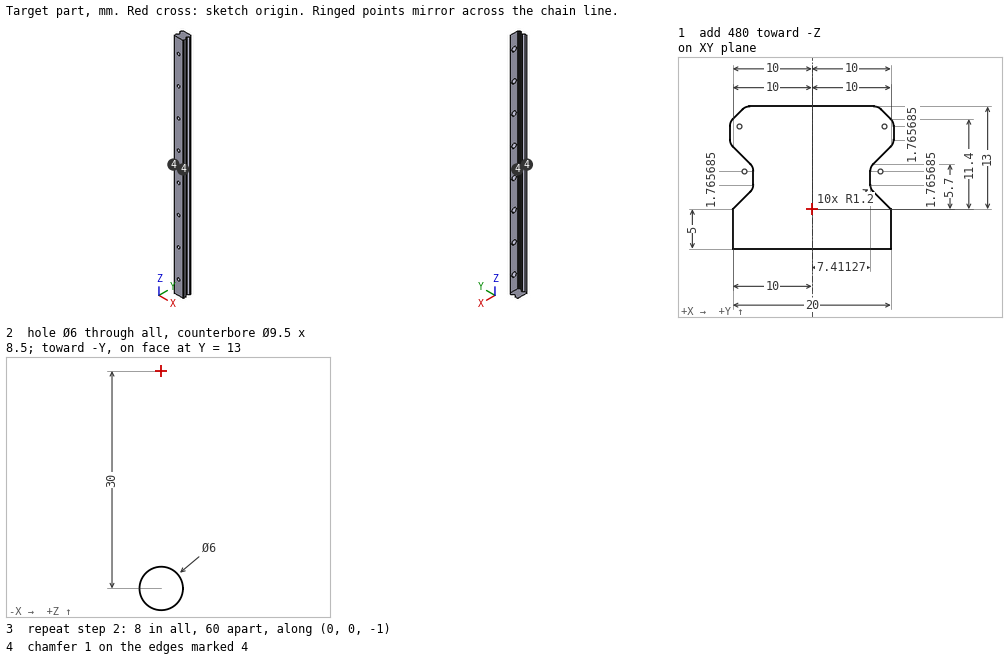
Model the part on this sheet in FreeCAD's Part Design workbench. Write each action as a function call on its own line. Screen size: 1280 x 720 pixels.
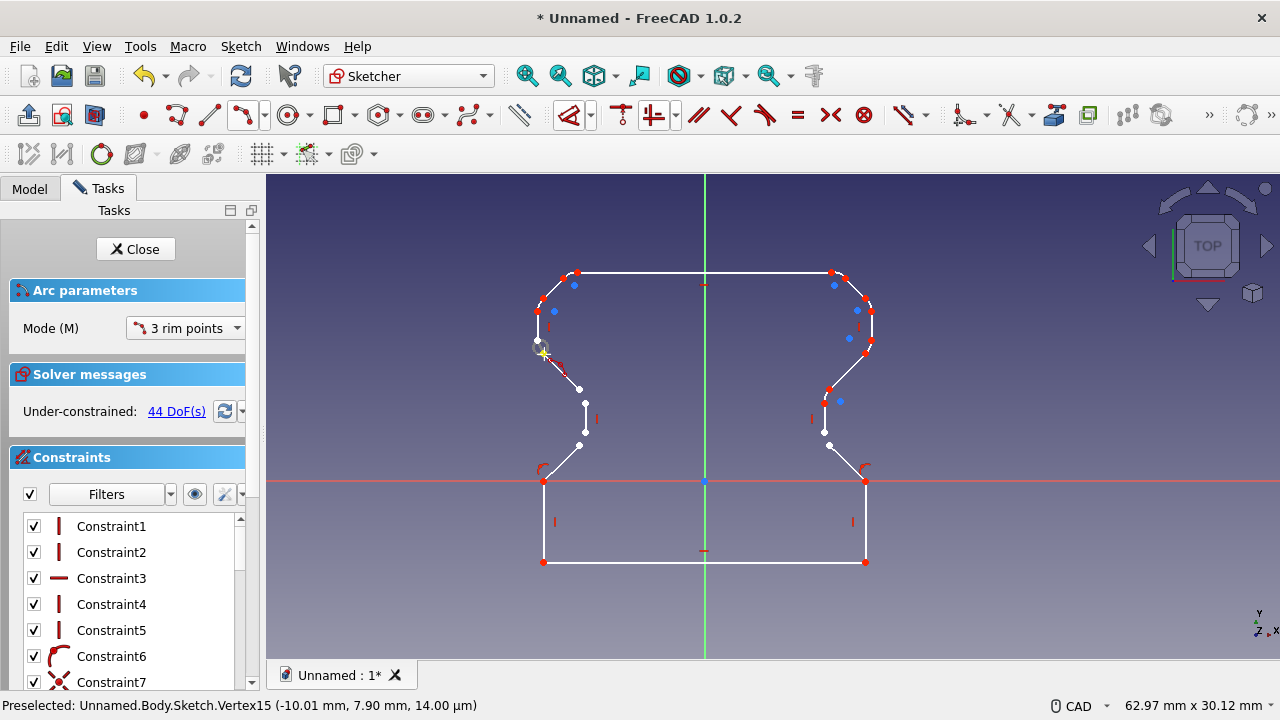
scroll(540, 347, up, 12)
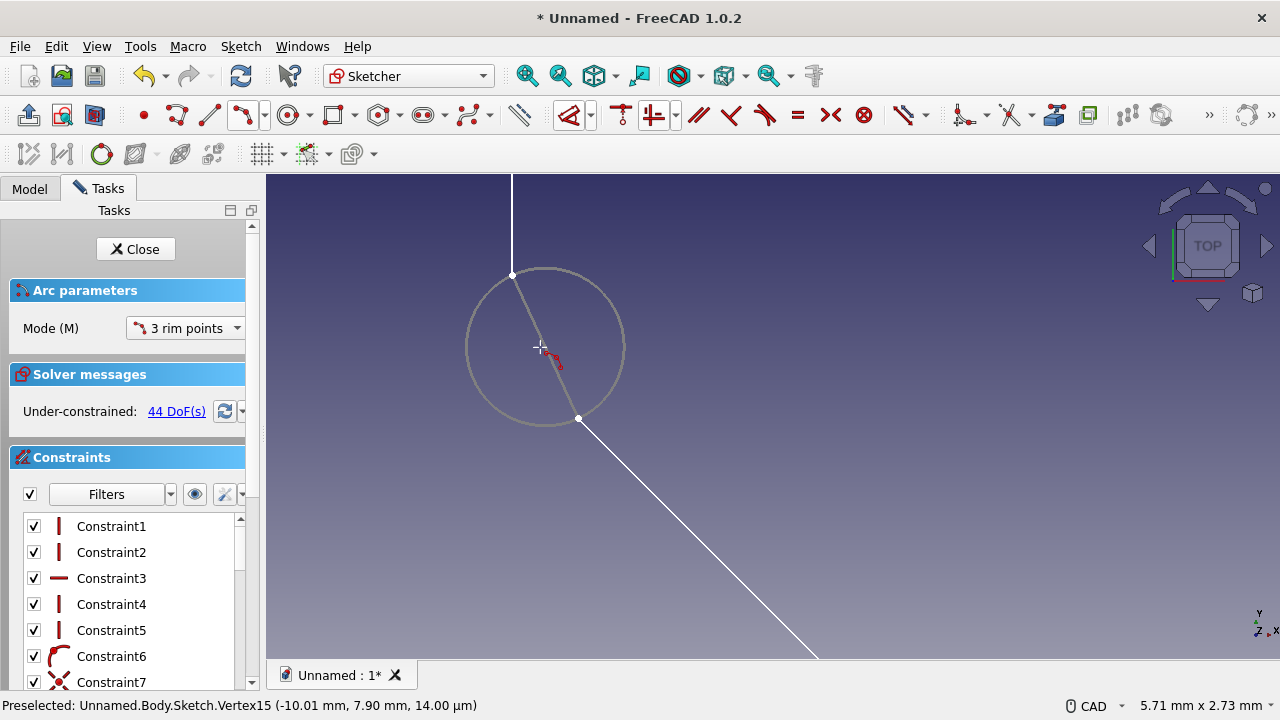
click(534, 344)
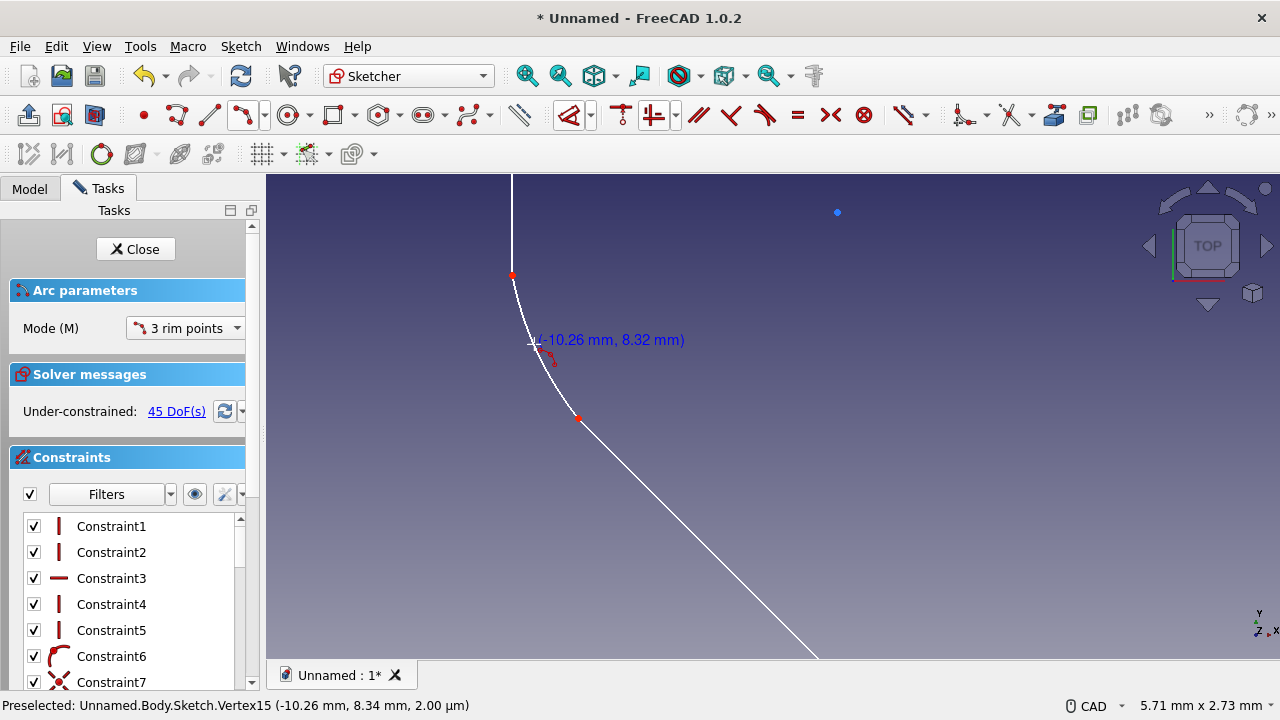
scroll(540, 347, down, 12)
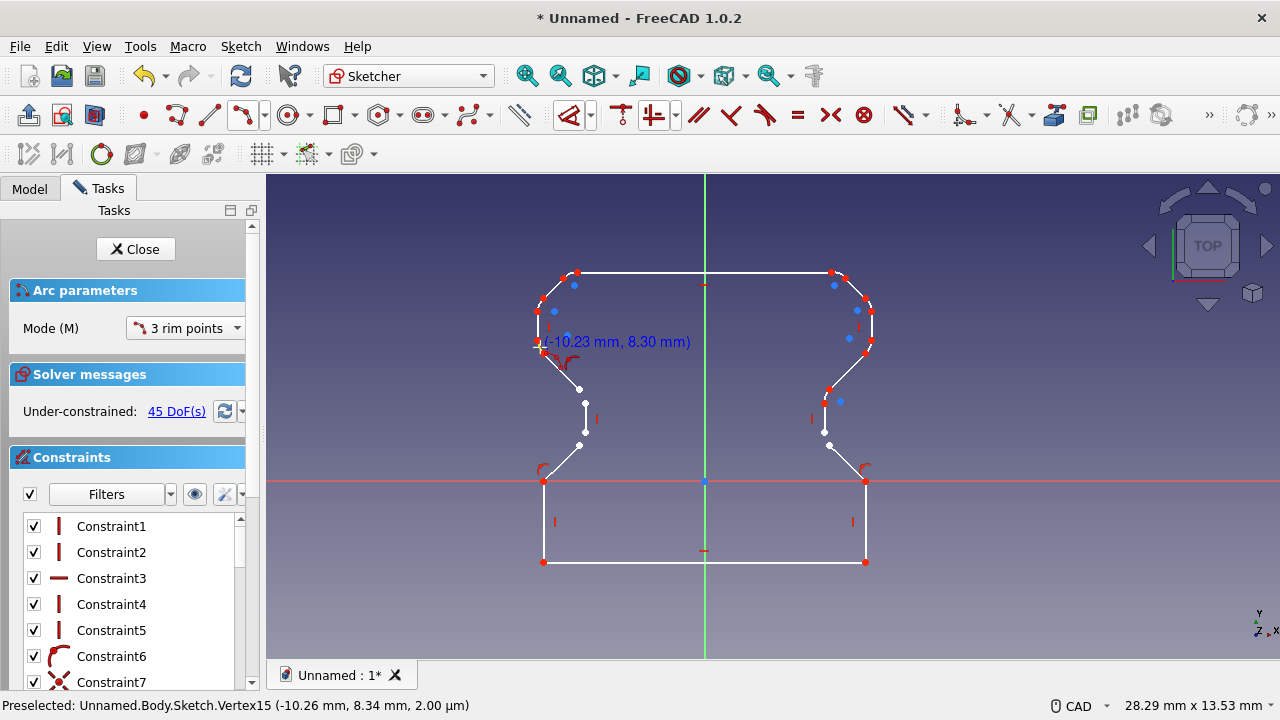
click(580, 390)
click(586, 404)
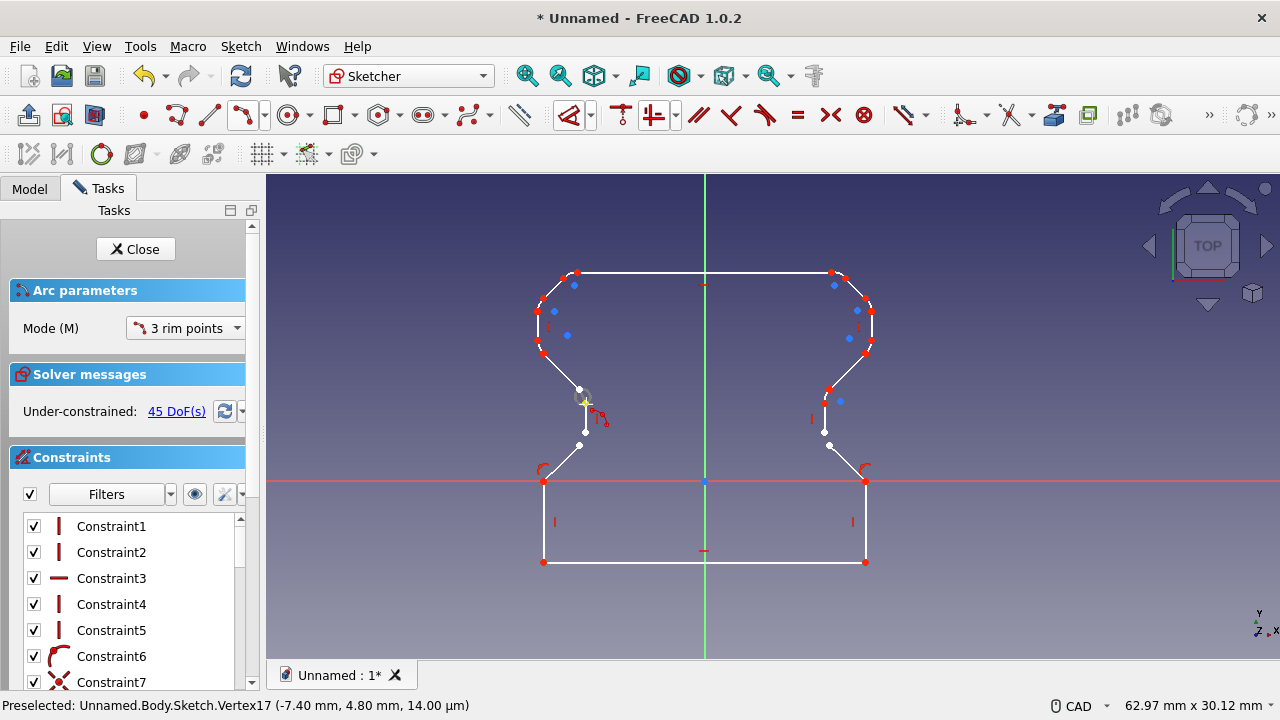
scroll(584, 396, up, 12)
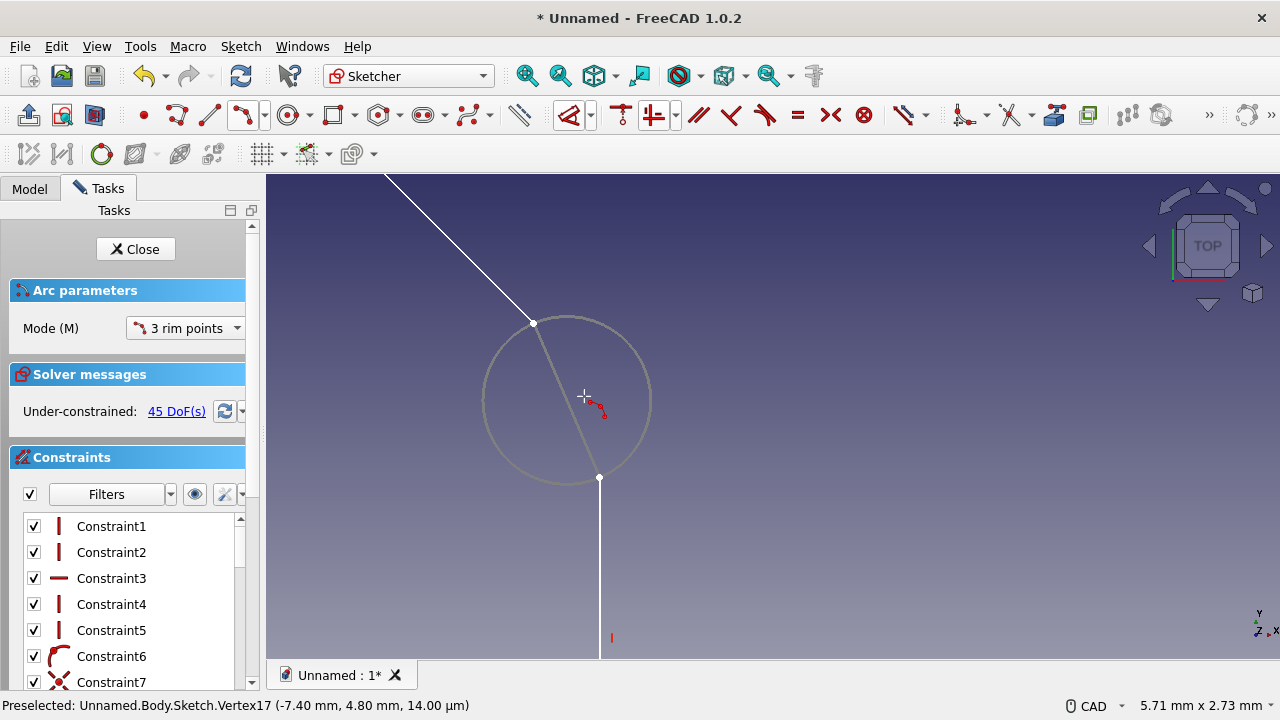
click(582, 387)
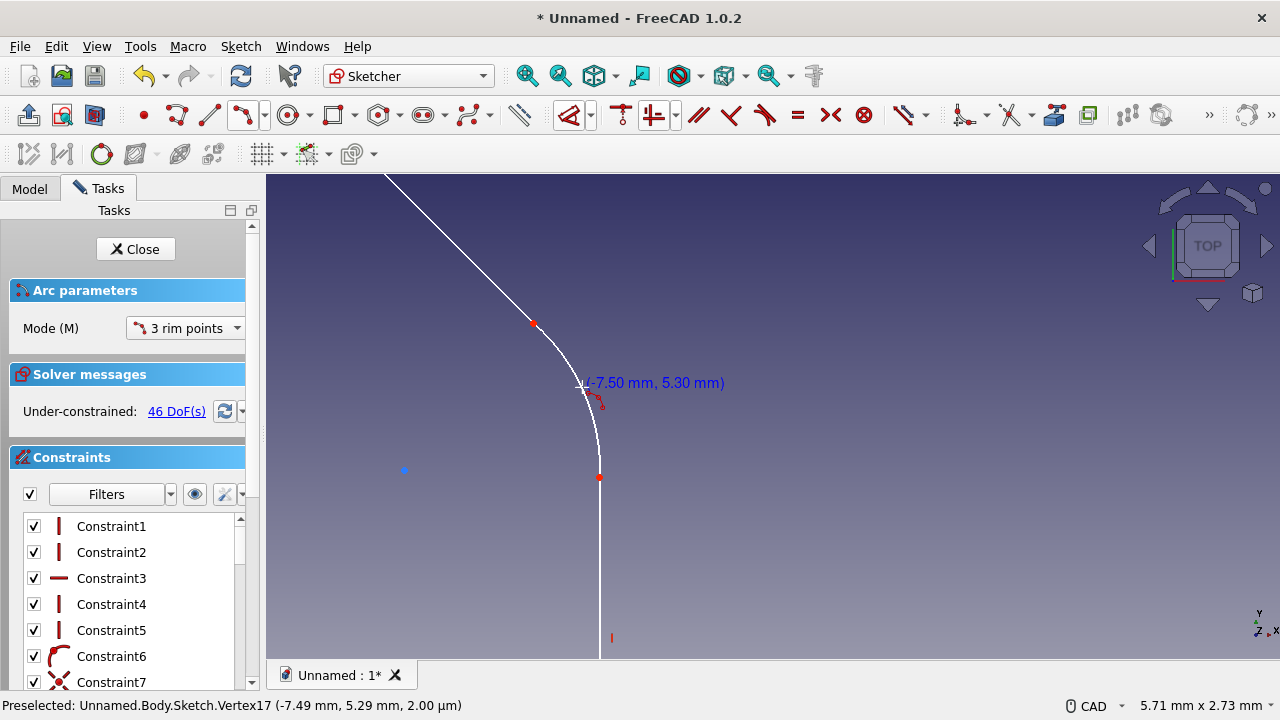
scroll(584, 396, down, 12)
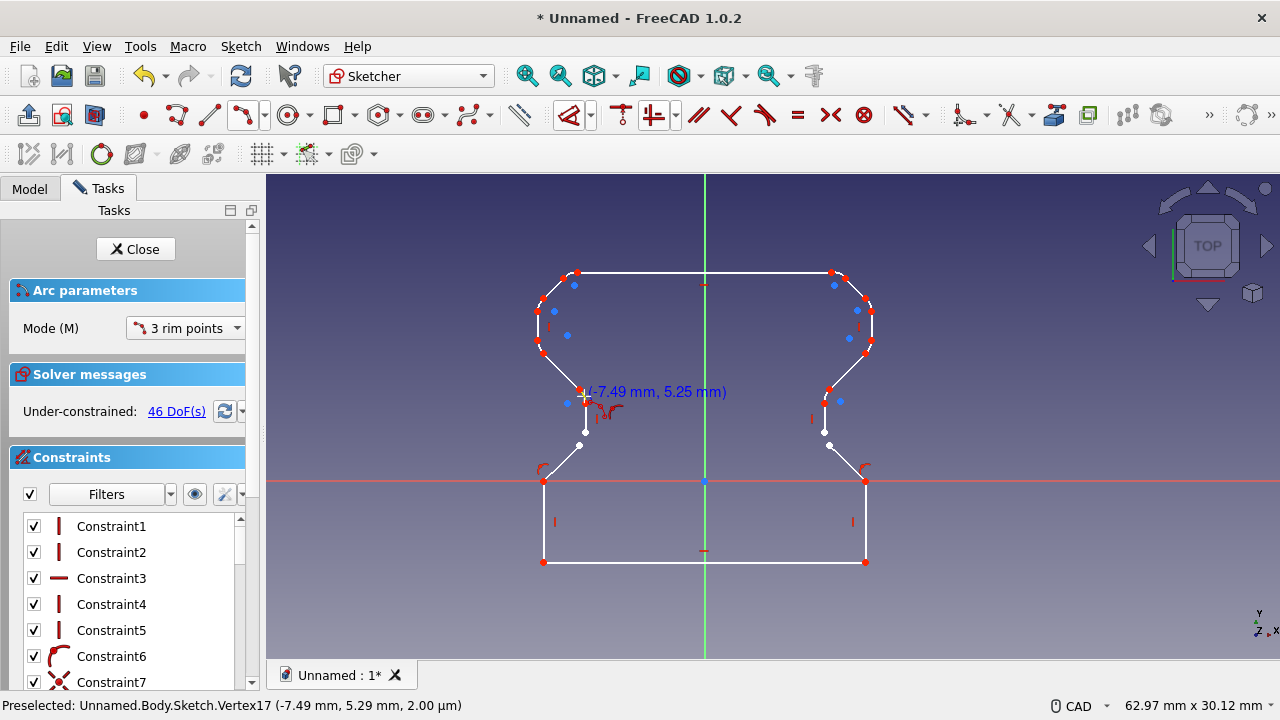
click(586, 433)
click(580, 446)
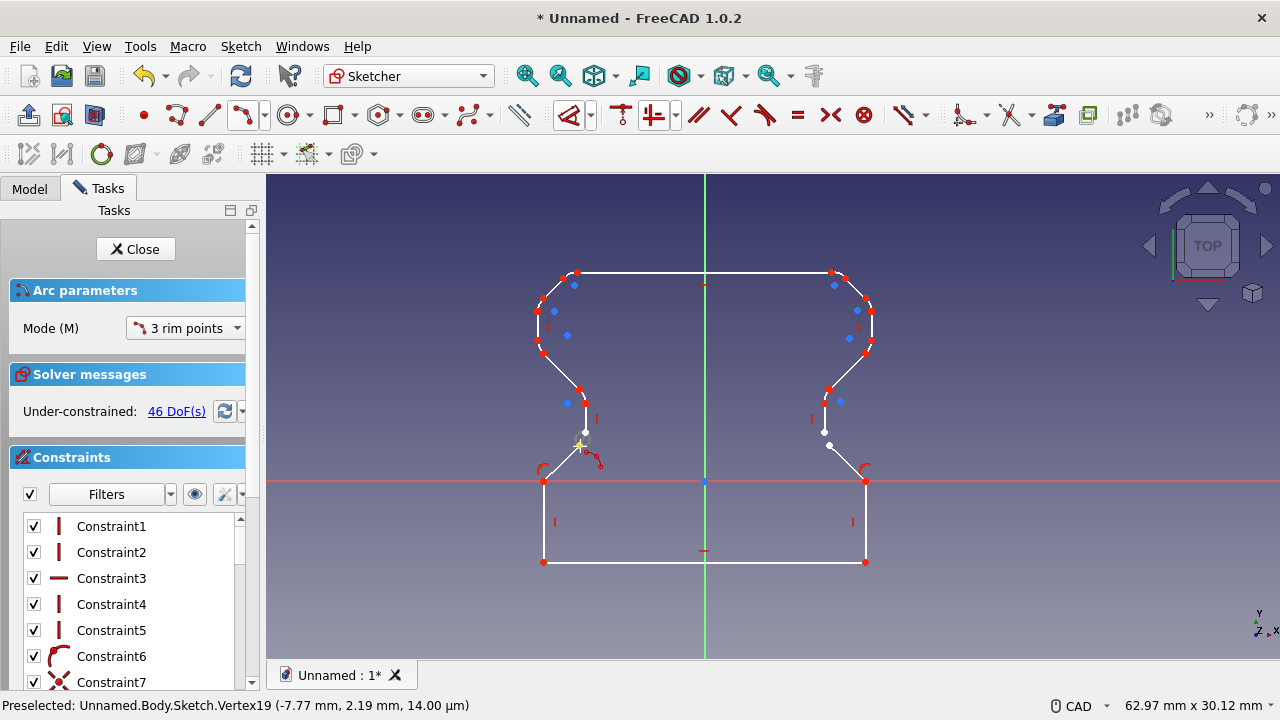
scroll(584, 439, up, 12)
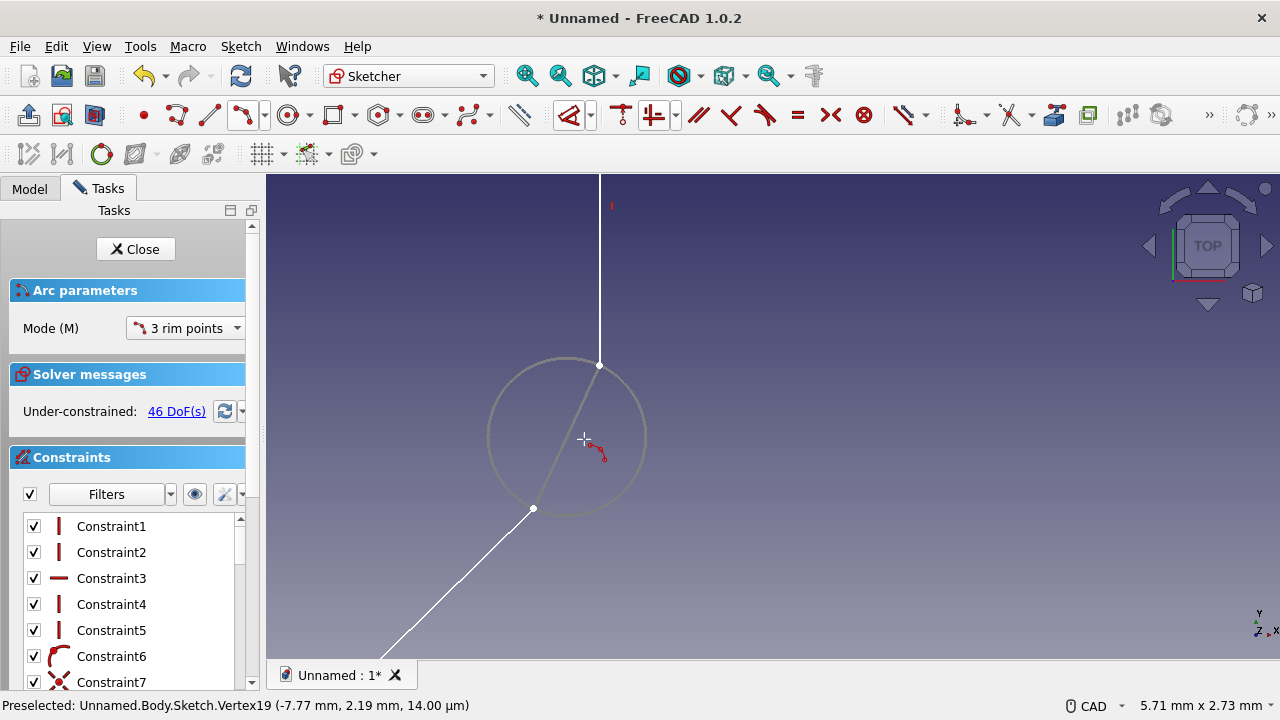
click(582, 431)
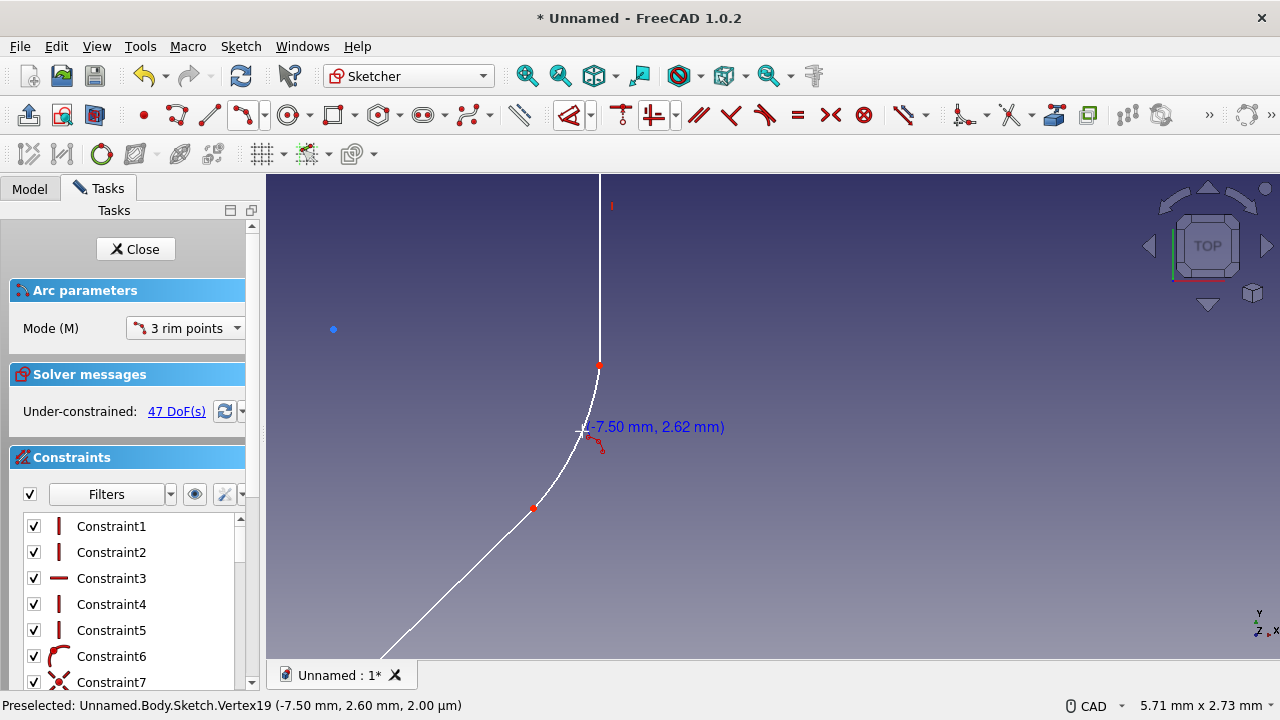
scroll(584, 439, down, 12)